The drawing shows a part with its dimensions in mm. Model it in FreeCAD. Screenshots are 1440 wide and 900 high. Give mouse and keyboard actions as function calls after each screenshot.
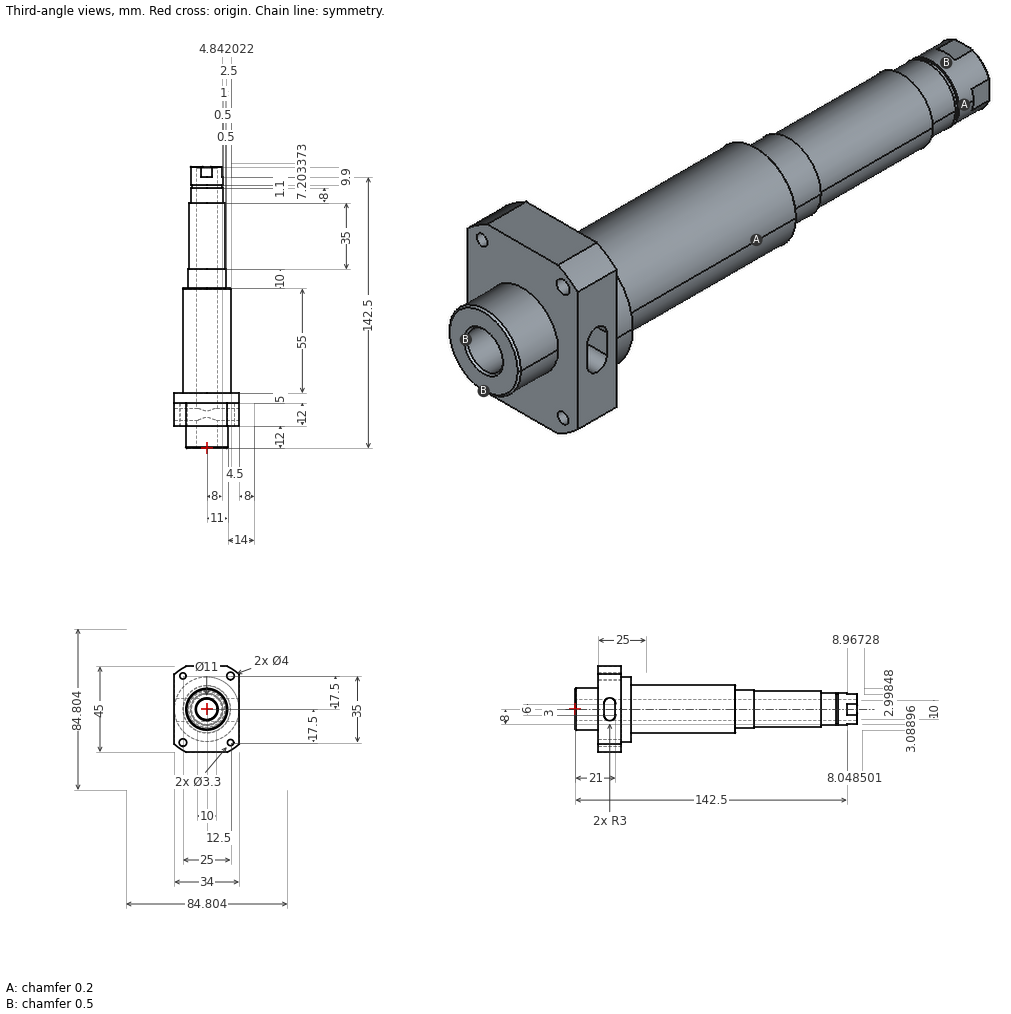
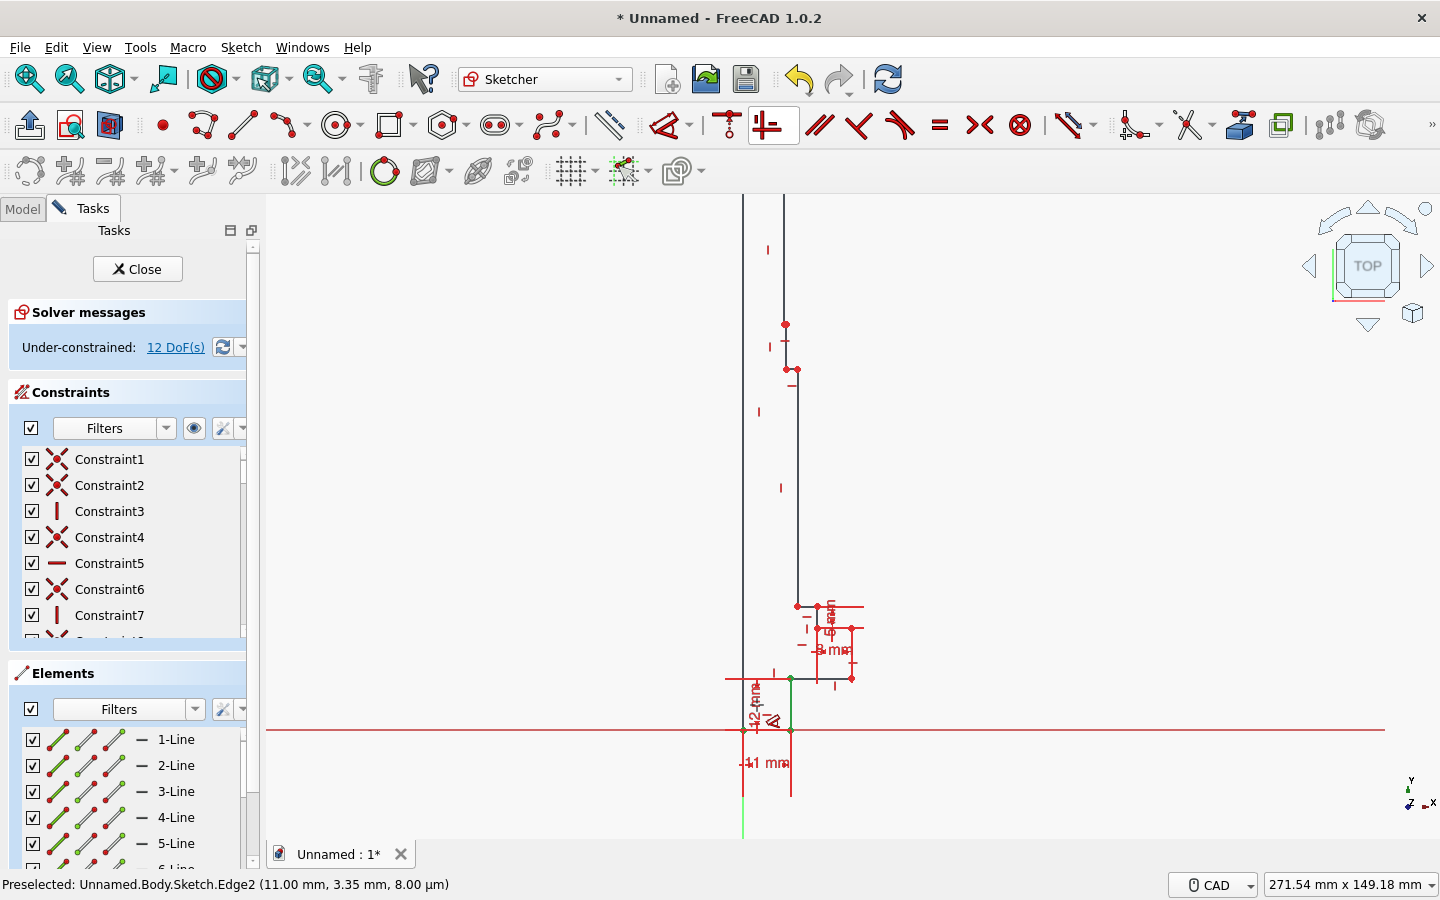
click(809, 679)
click(835, 713)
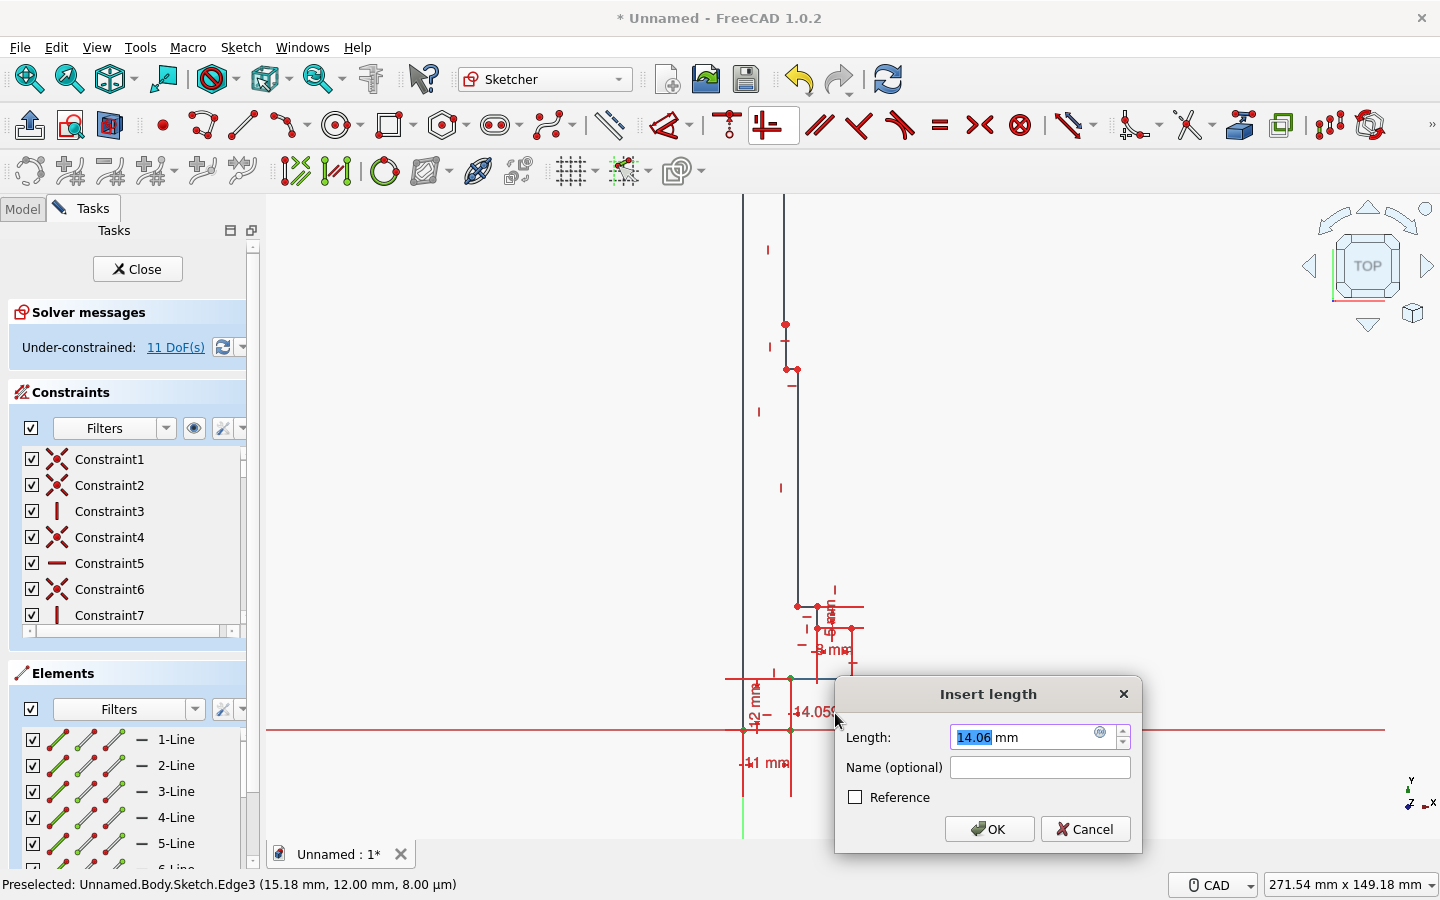
text(14)
key(Return)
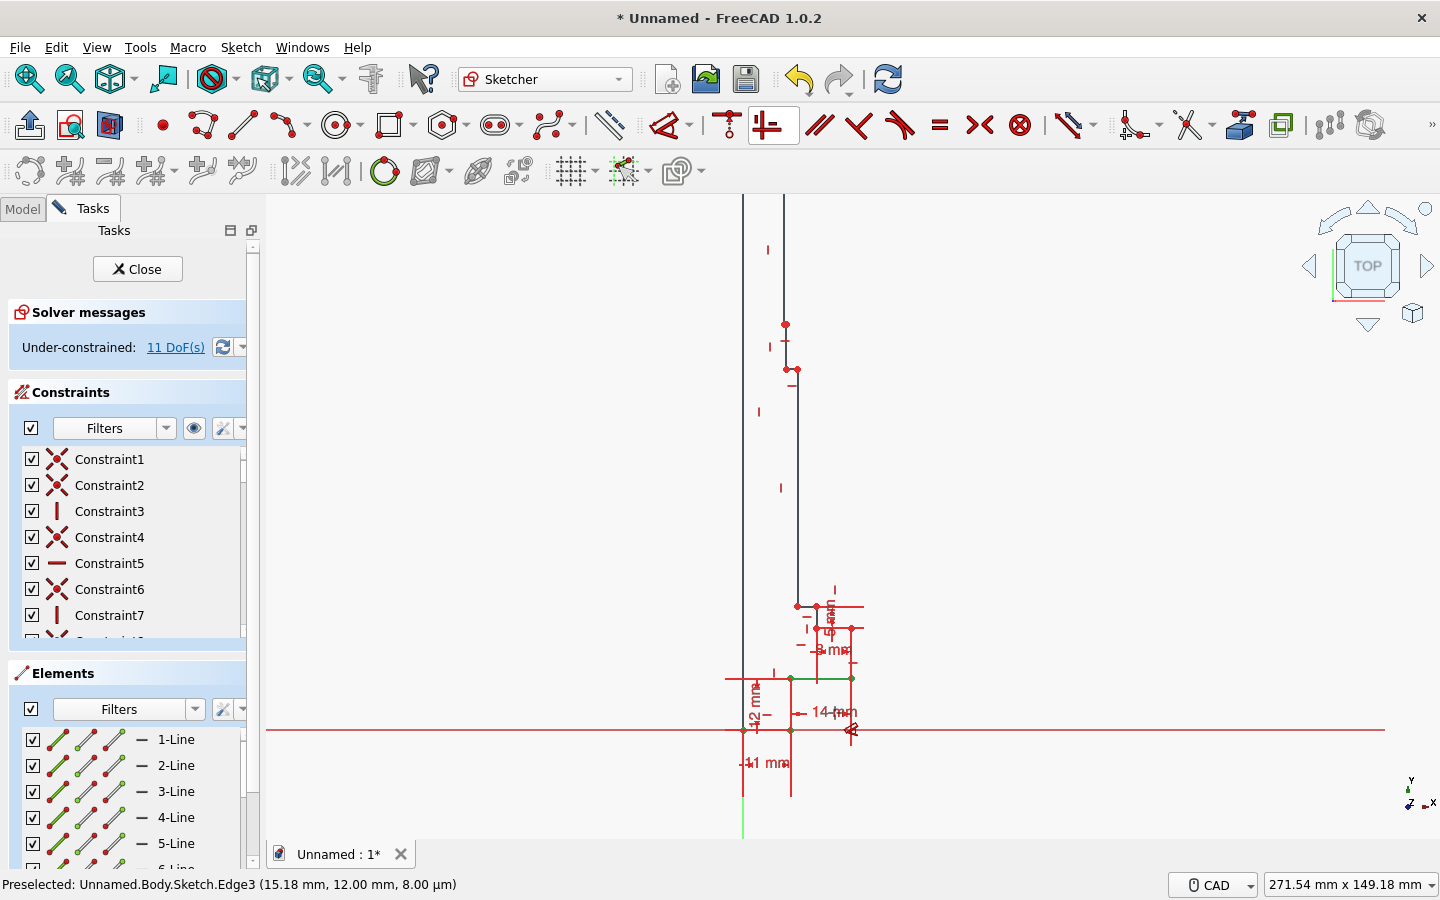
click(851, 664)
click(909, 654)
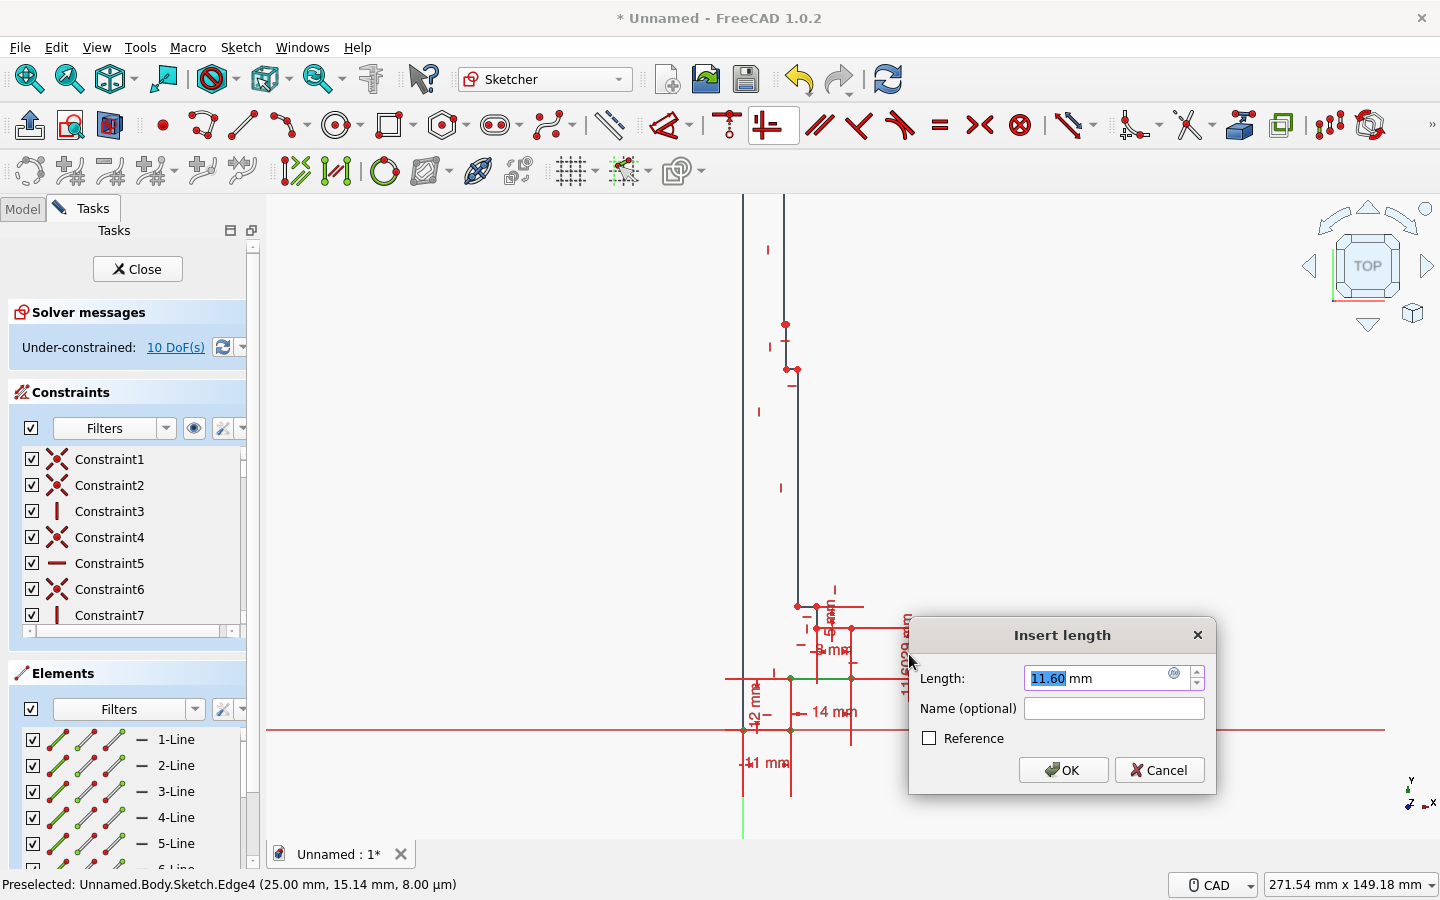
text(12)
key(Return)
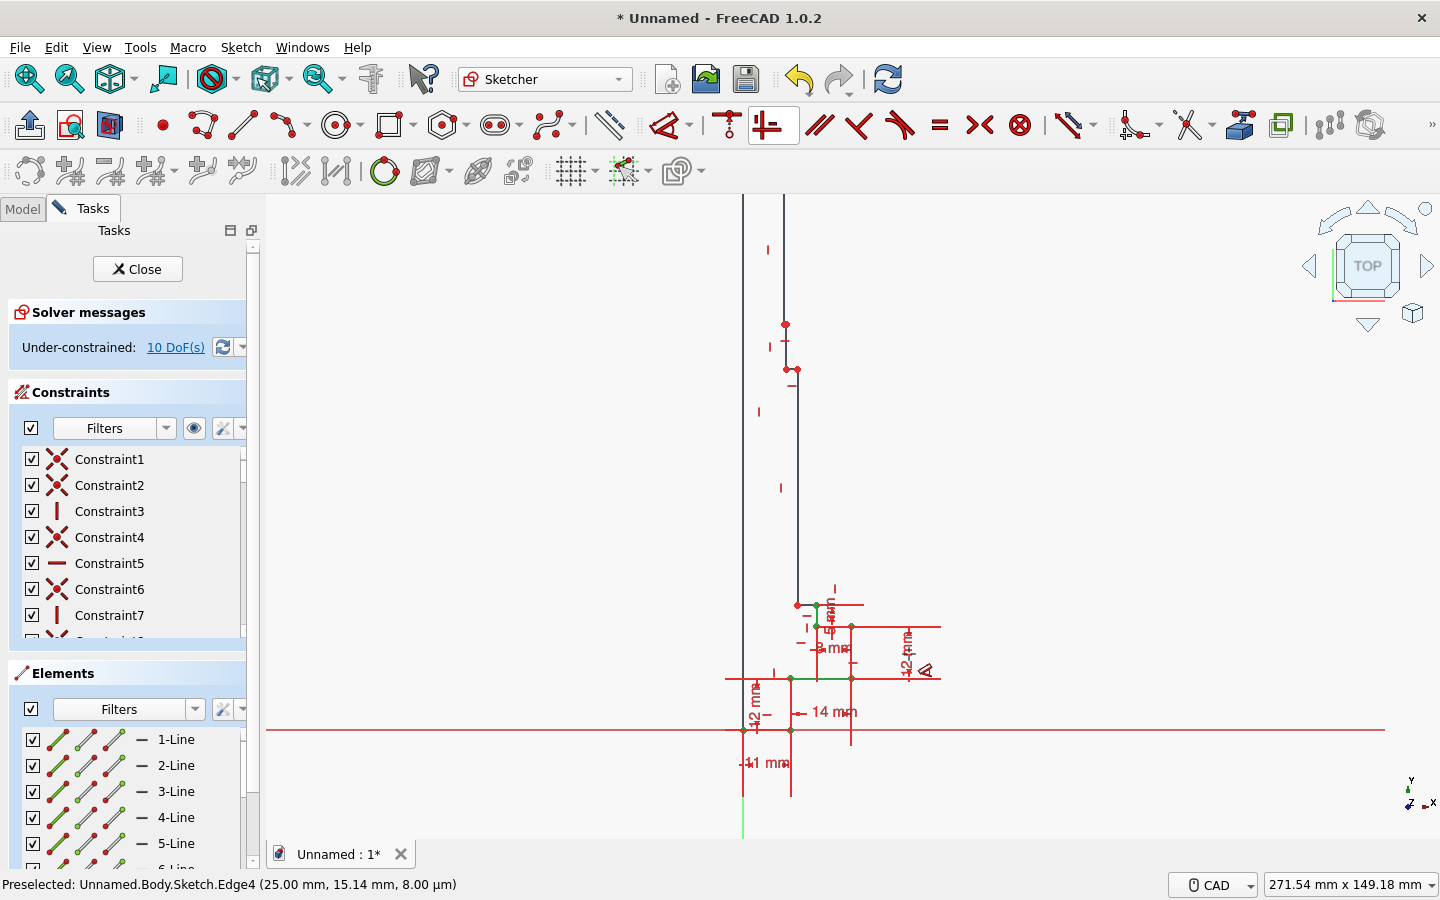
click(798, 534)
click(832, 487)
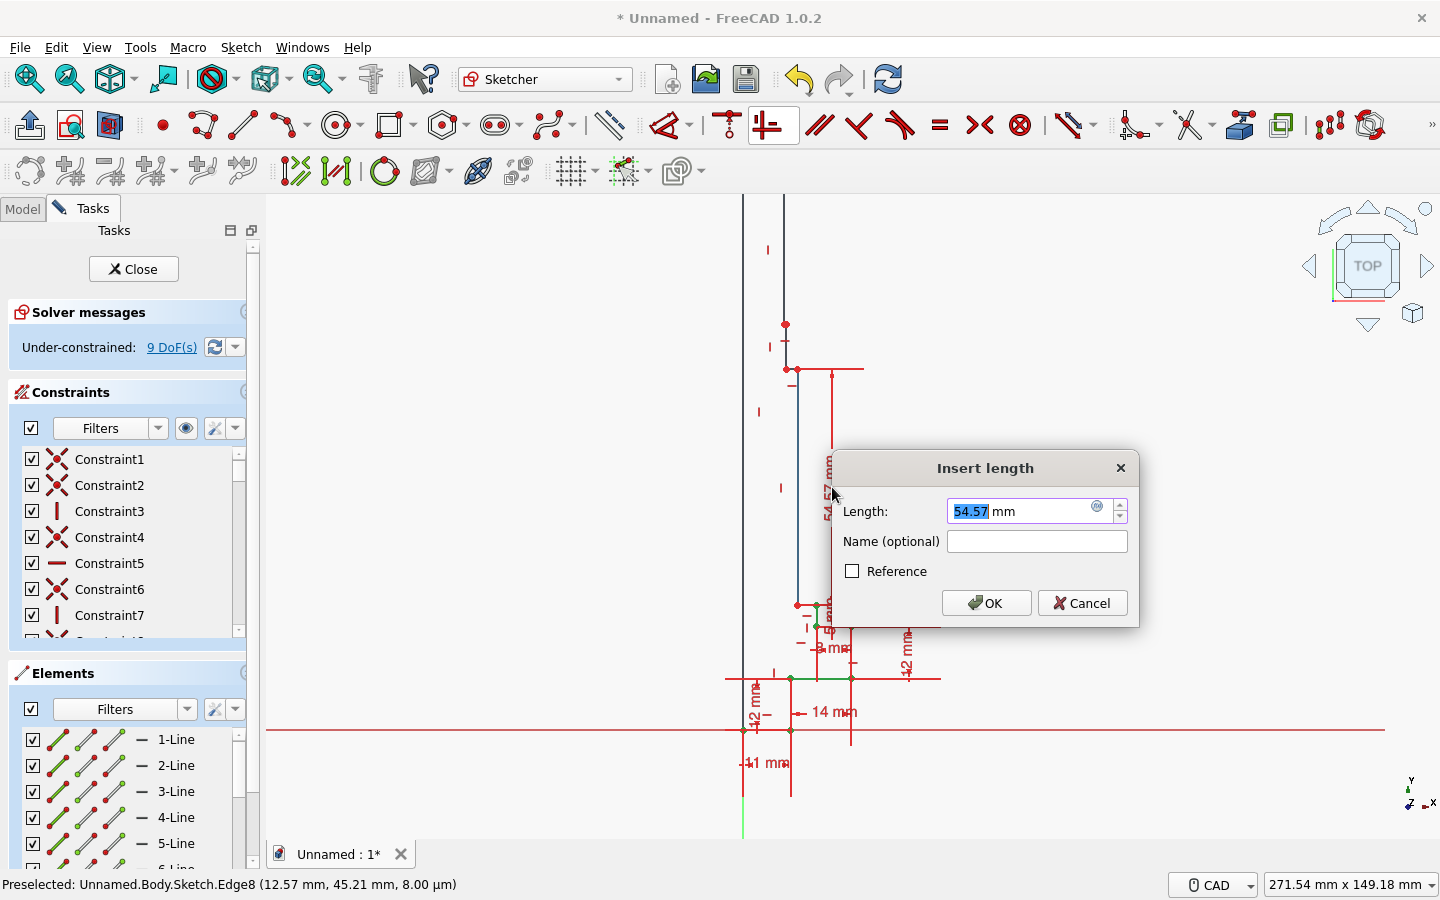
text(55)
key(Return)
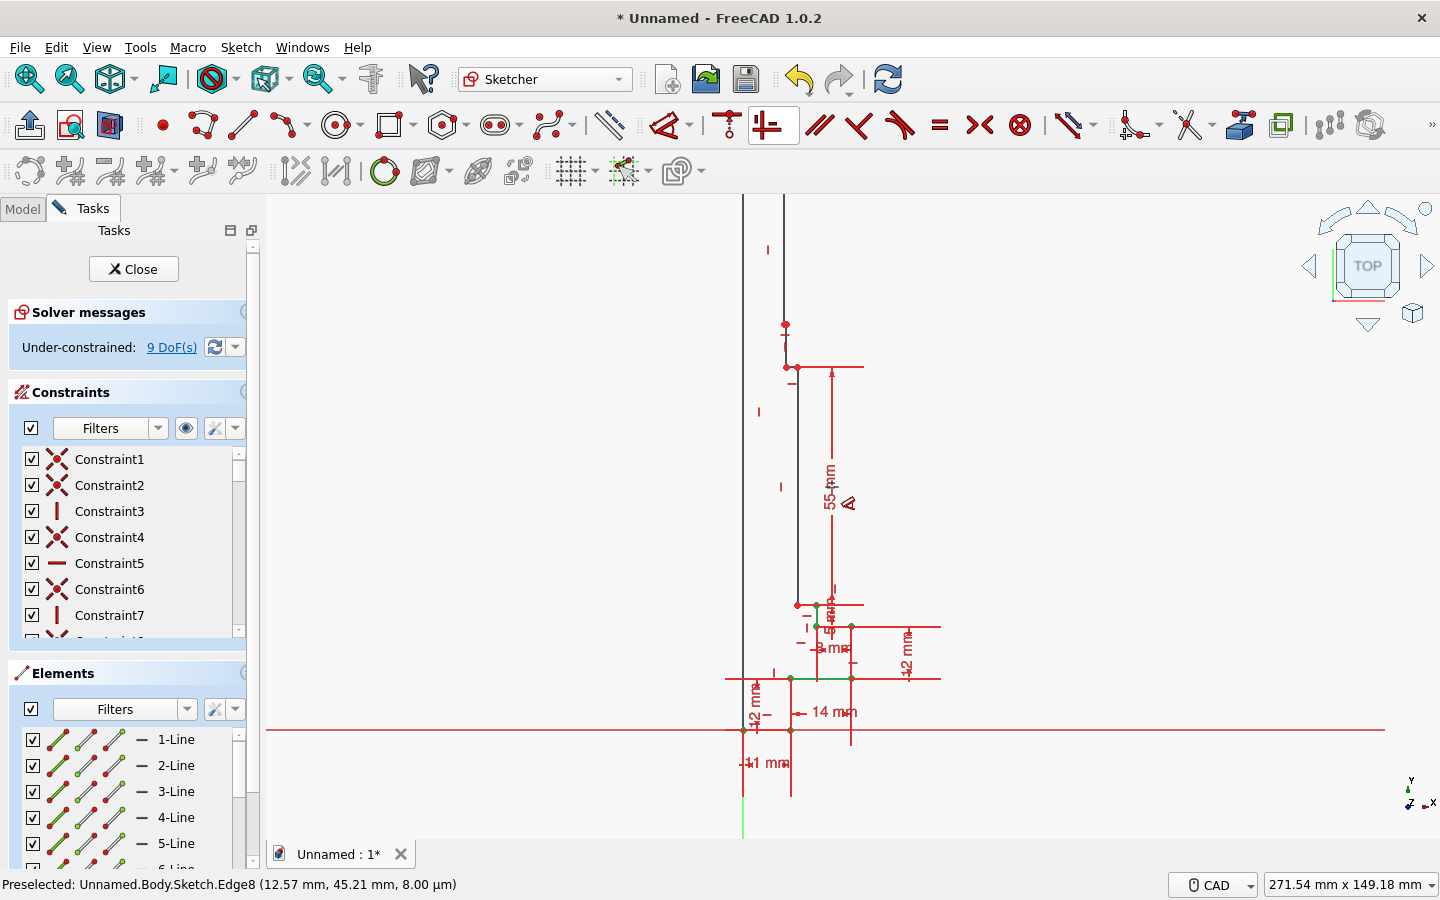
click(786, 354)
click(820, 346)